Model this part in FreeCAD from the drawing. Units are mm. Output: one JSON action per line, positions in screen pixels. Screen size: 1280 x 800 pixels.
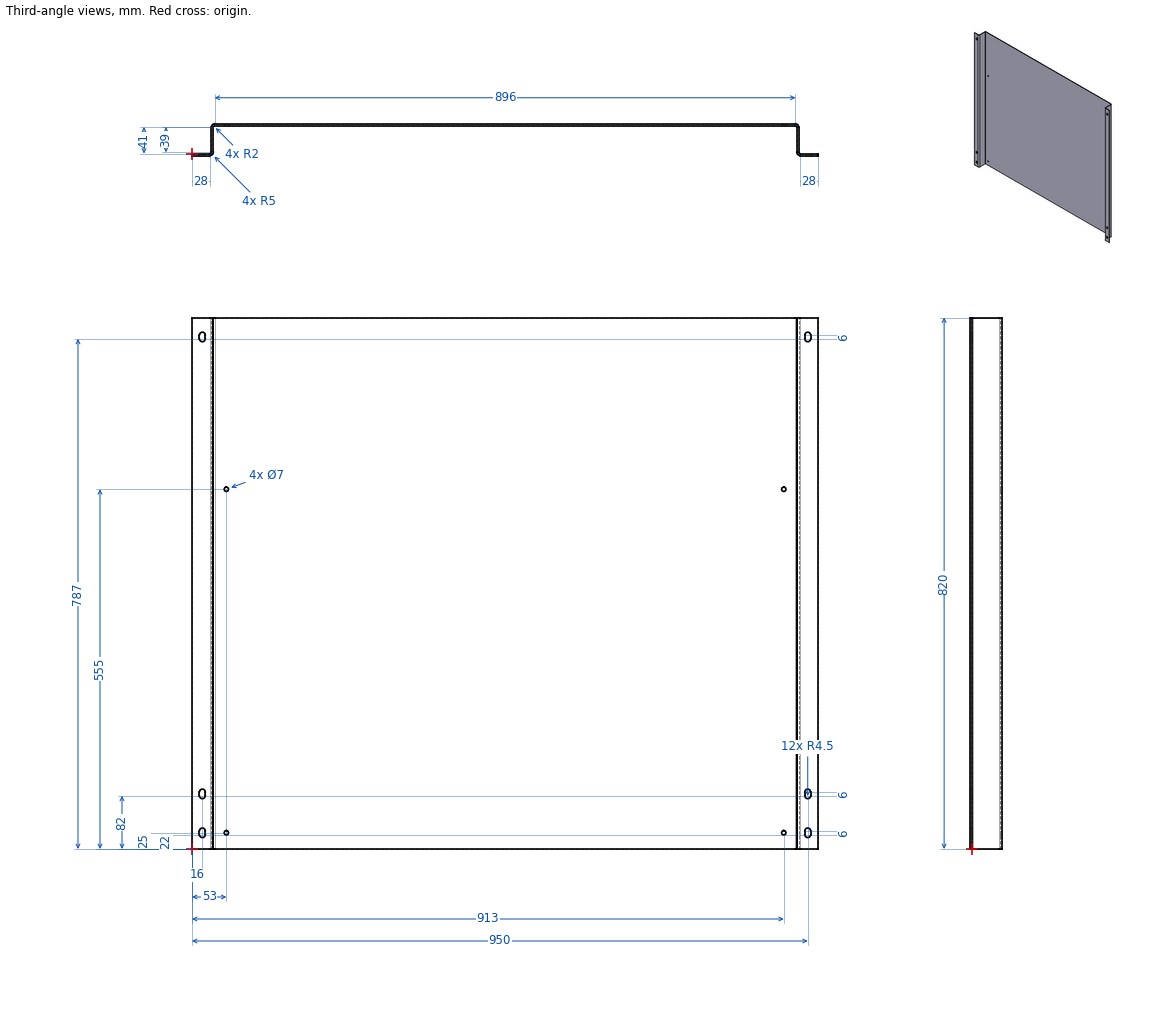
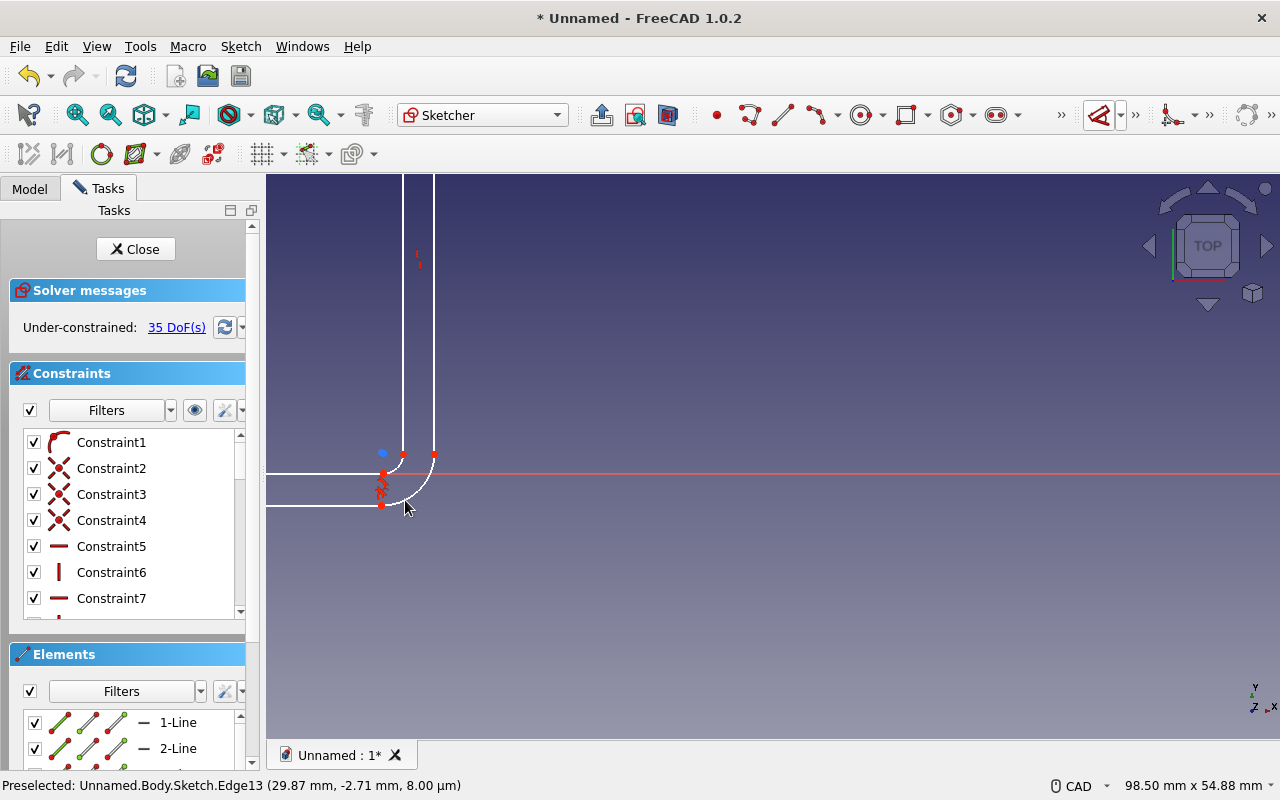
{"action": "left_click", "coordinate": [434, 341]}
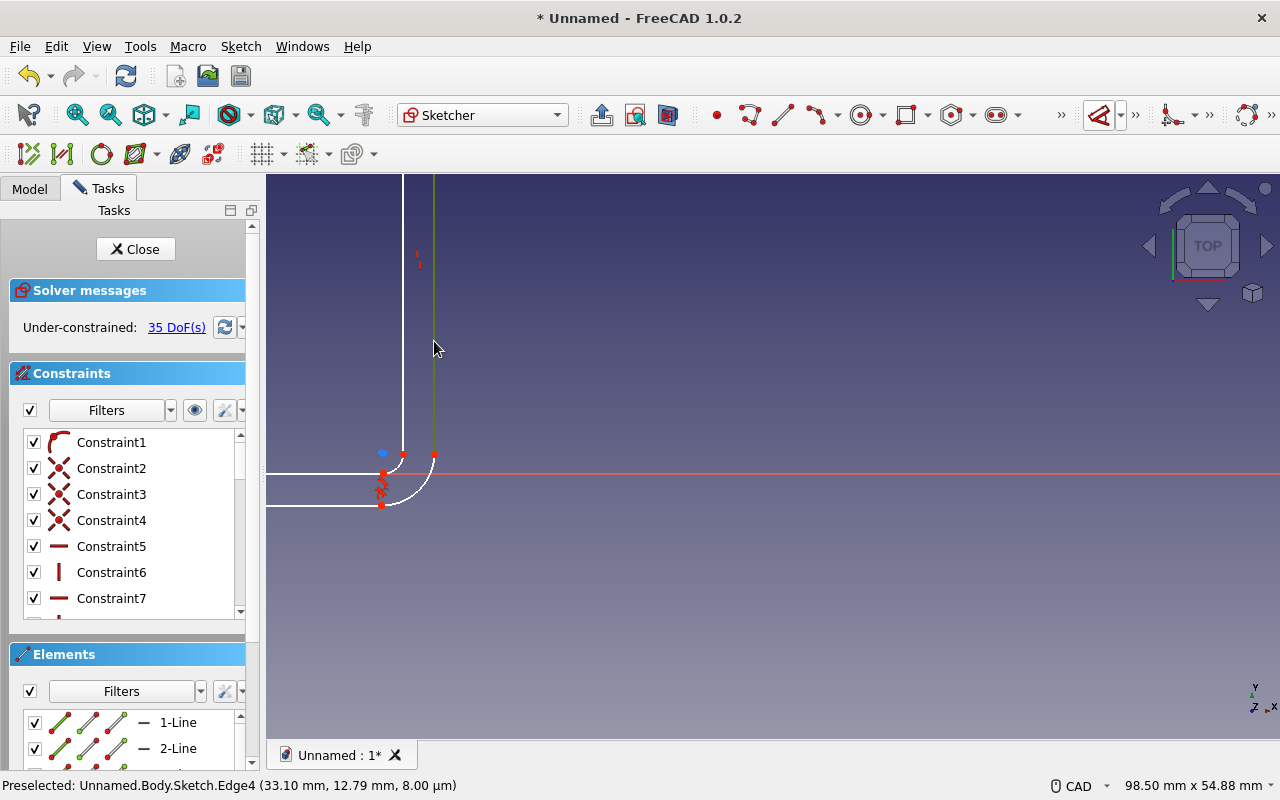
{"action": "left_click", "coordinate": [405, 500]}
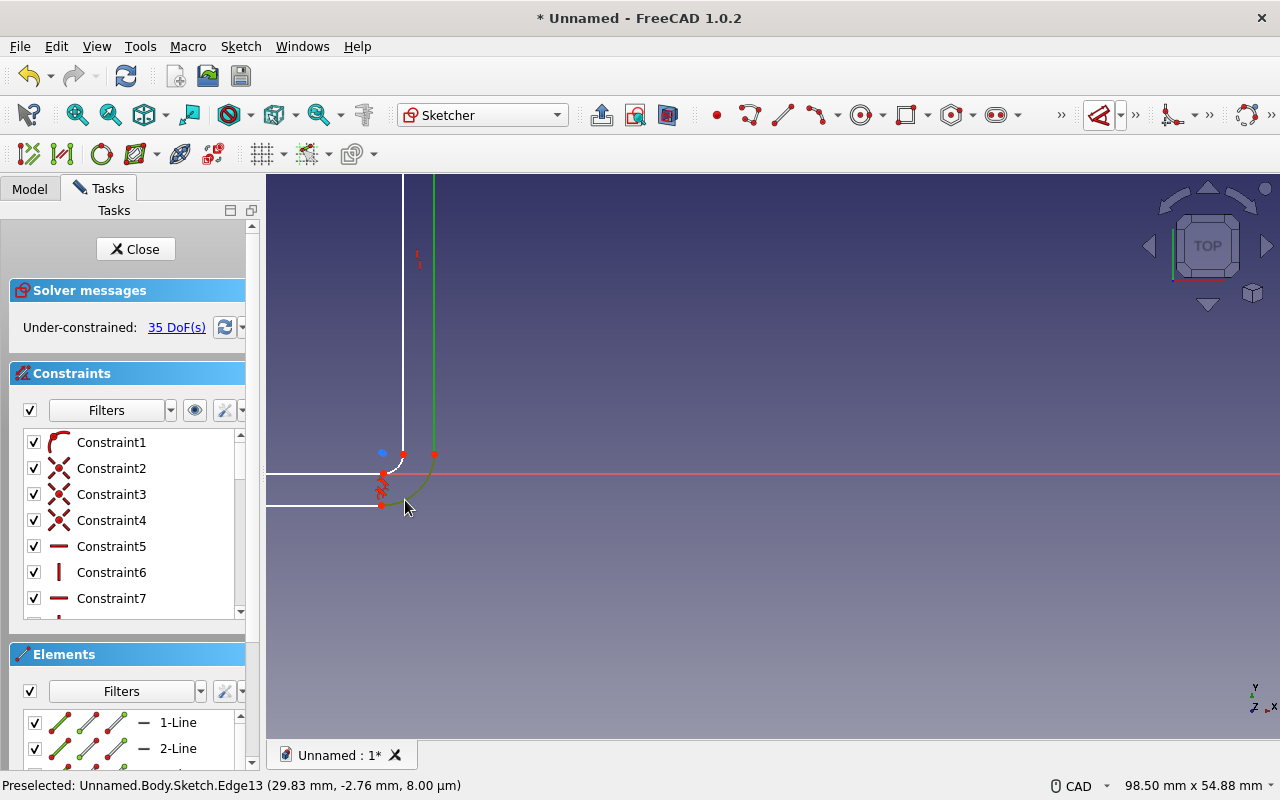
{"action": "key", "text": "t"}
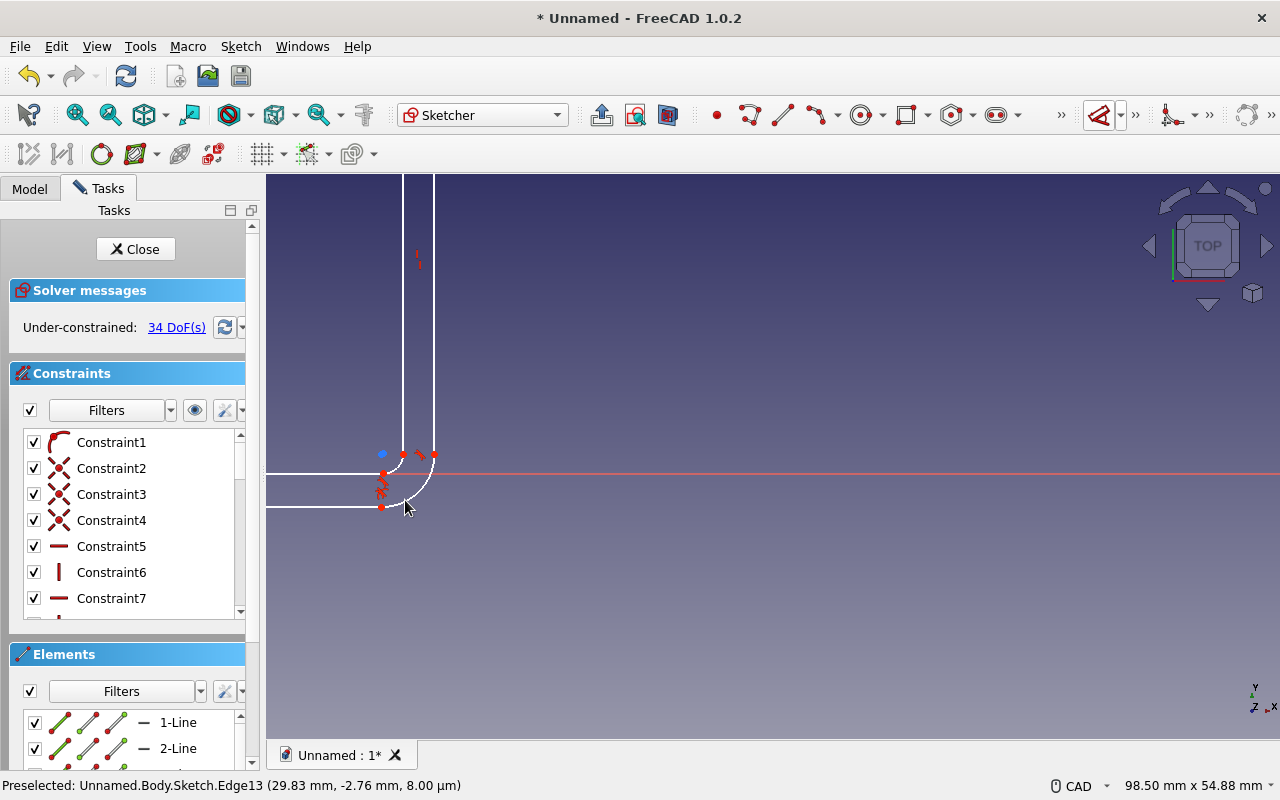
{"action": "left_click", "coordinate": [434, 341]}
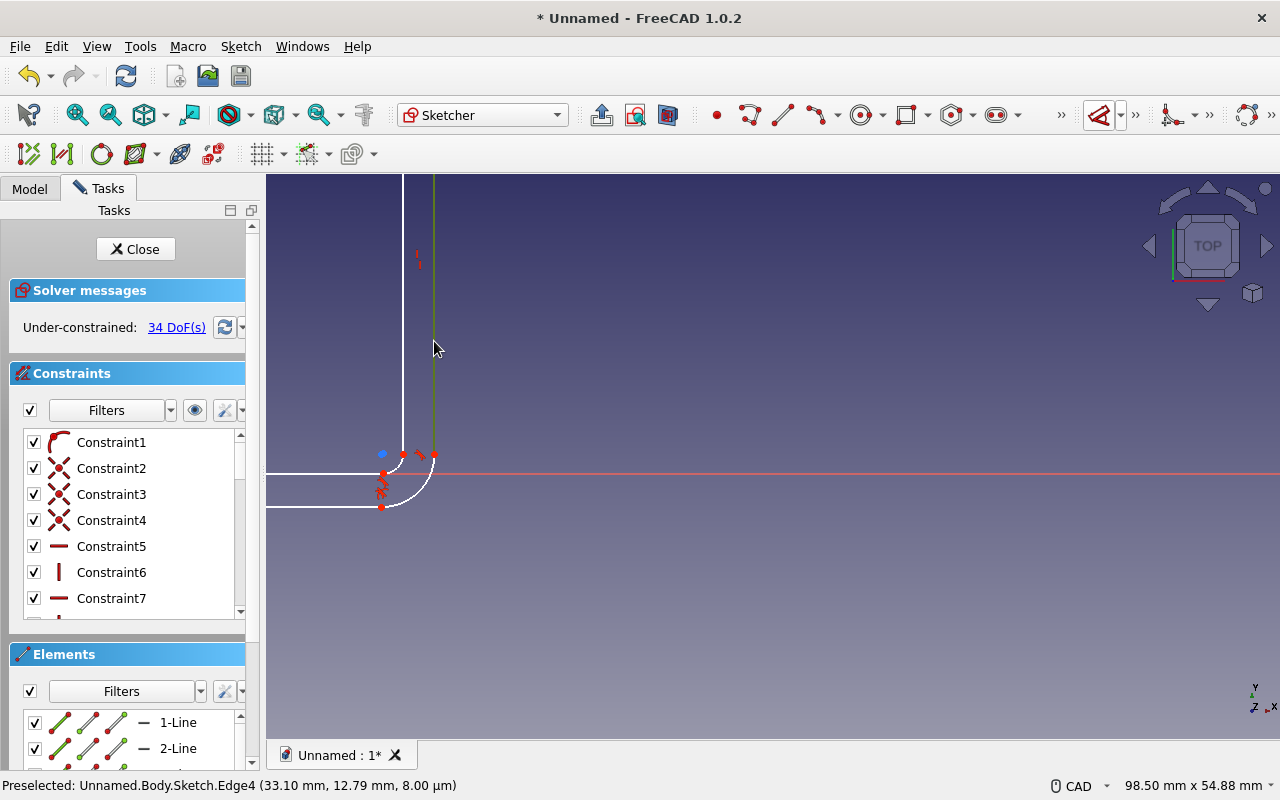
{"action": "scroll", "coordinate": [422, 470], "scroll_direction": "down", "scroll_amount": 14}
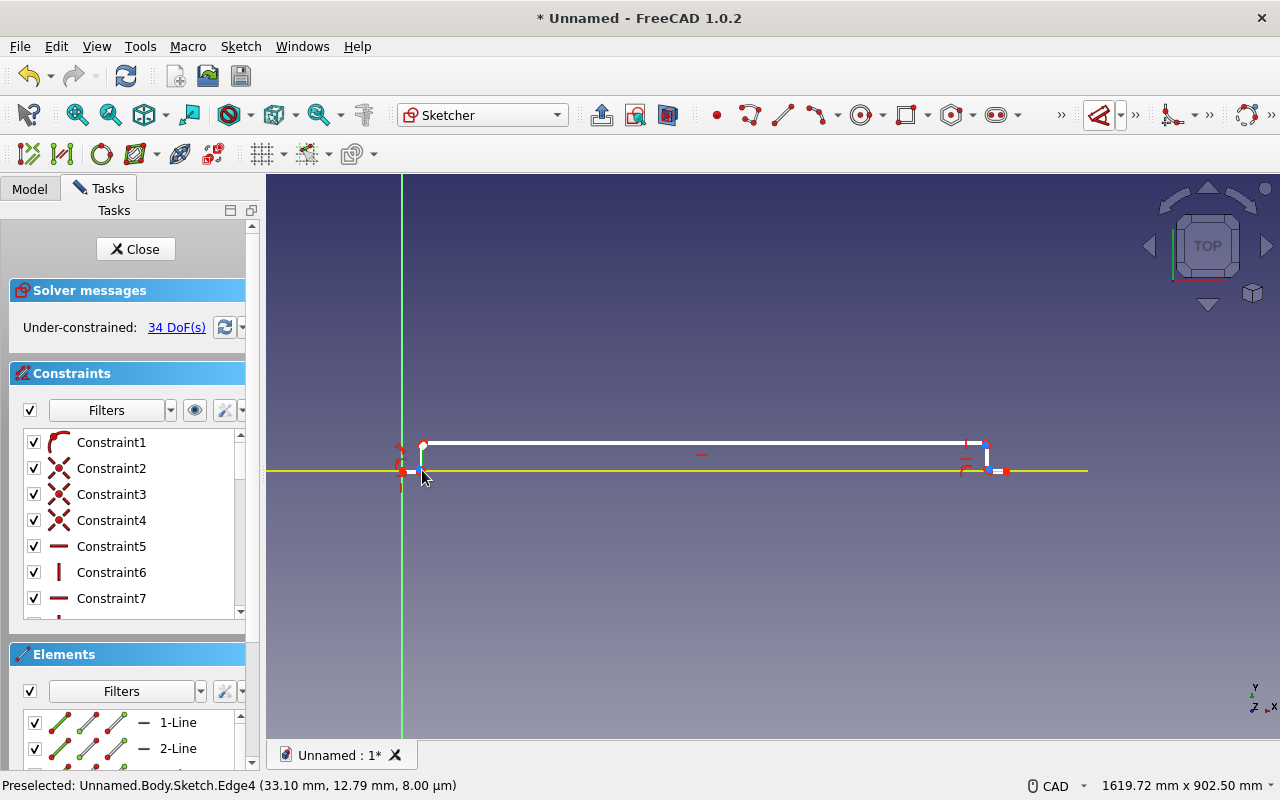
{"action": "scroll", "coordinate": [423, 444], "scroll_direction": "up", "scroll_amount": 14}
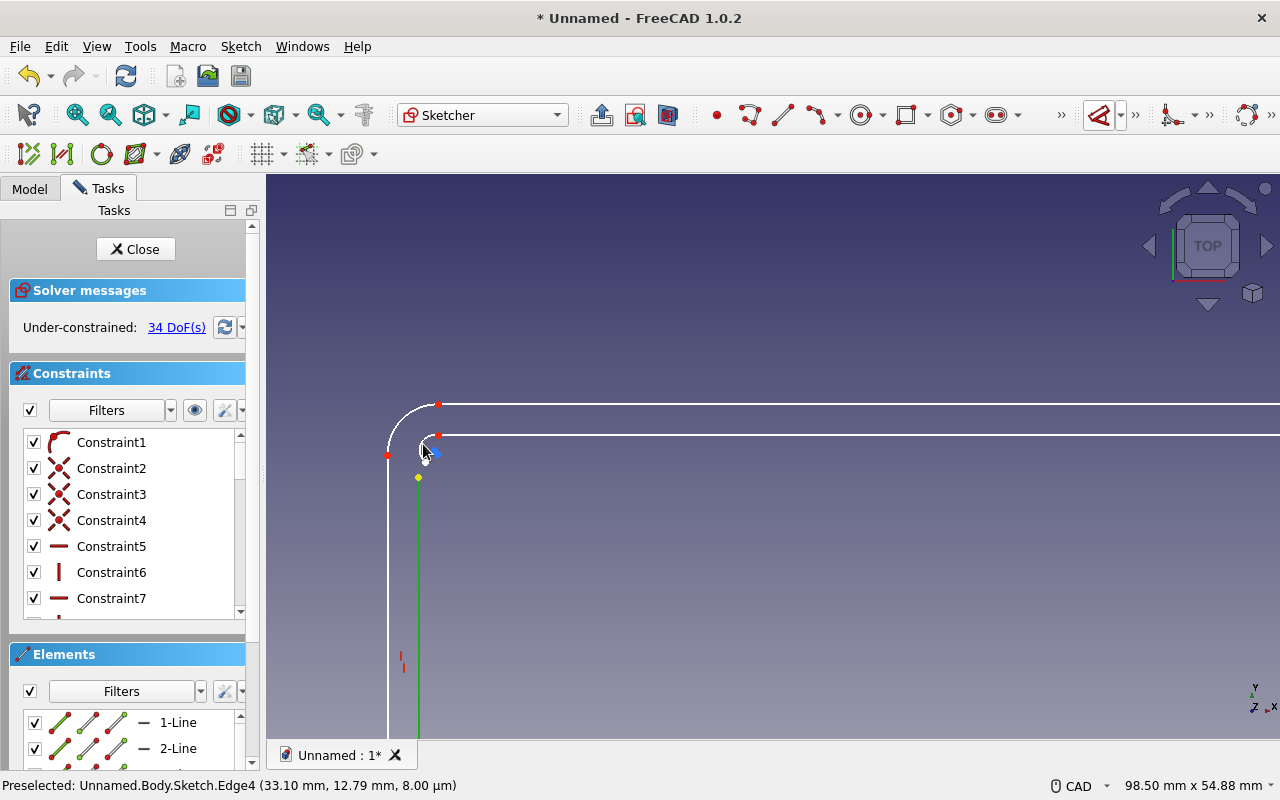
{"action": "left_click", "coordinate": [426, 438]}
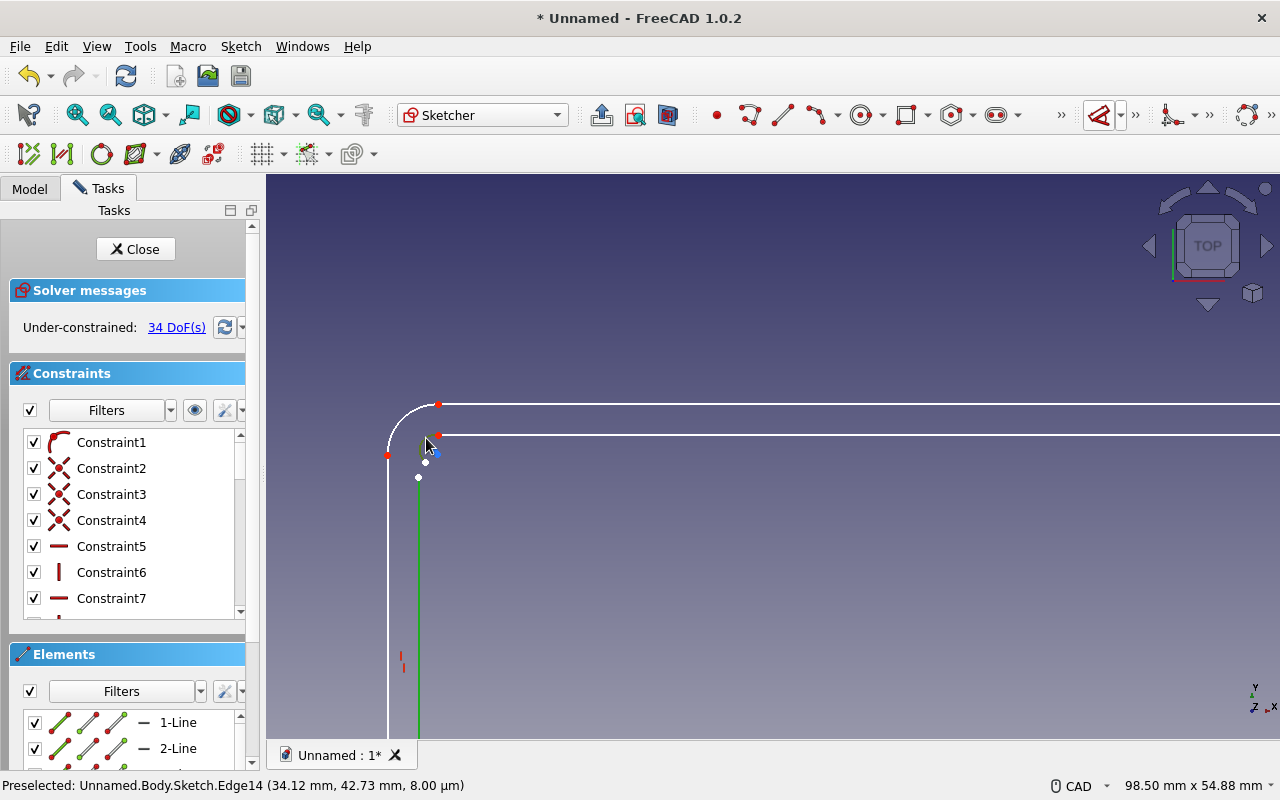
{"action": "key", "text": "t"}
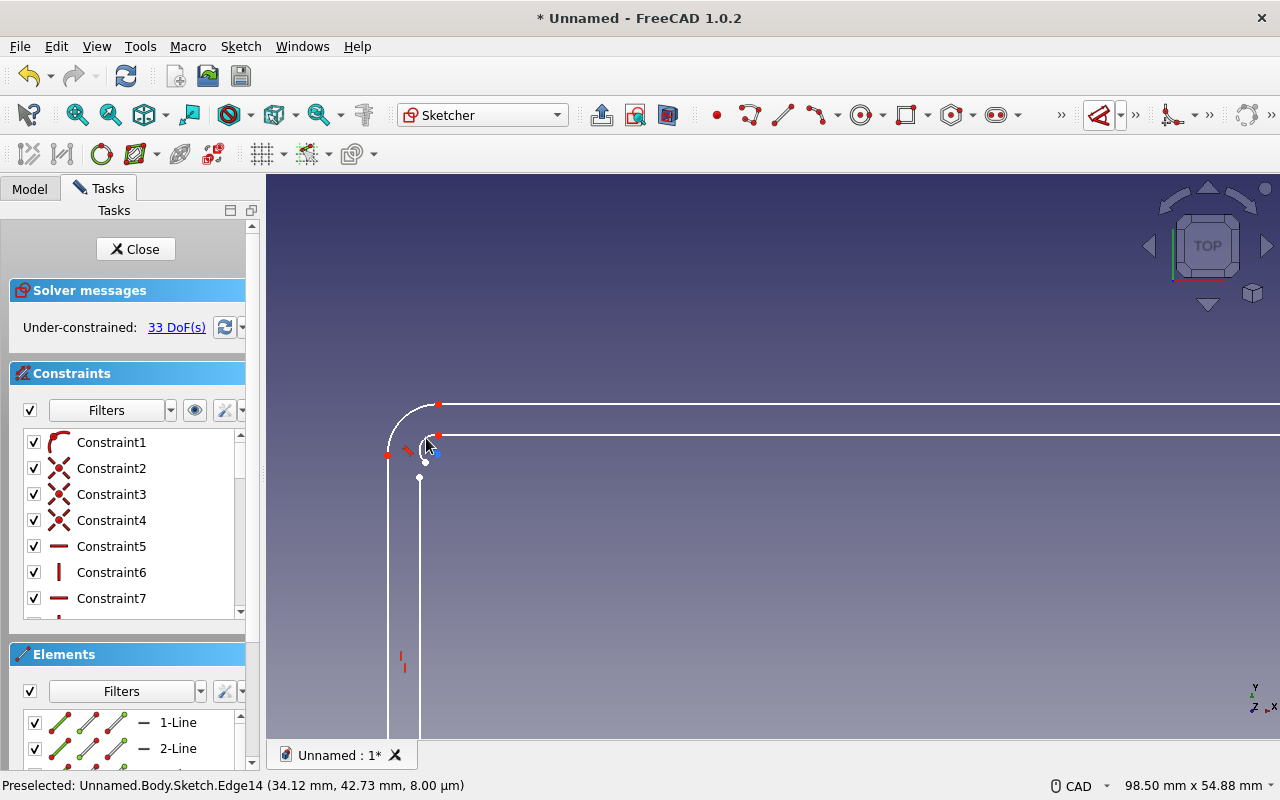
{"action": "scroll", "coordinate": [423, 444], "scroll_direction": "down", "scroll_amount": 14}